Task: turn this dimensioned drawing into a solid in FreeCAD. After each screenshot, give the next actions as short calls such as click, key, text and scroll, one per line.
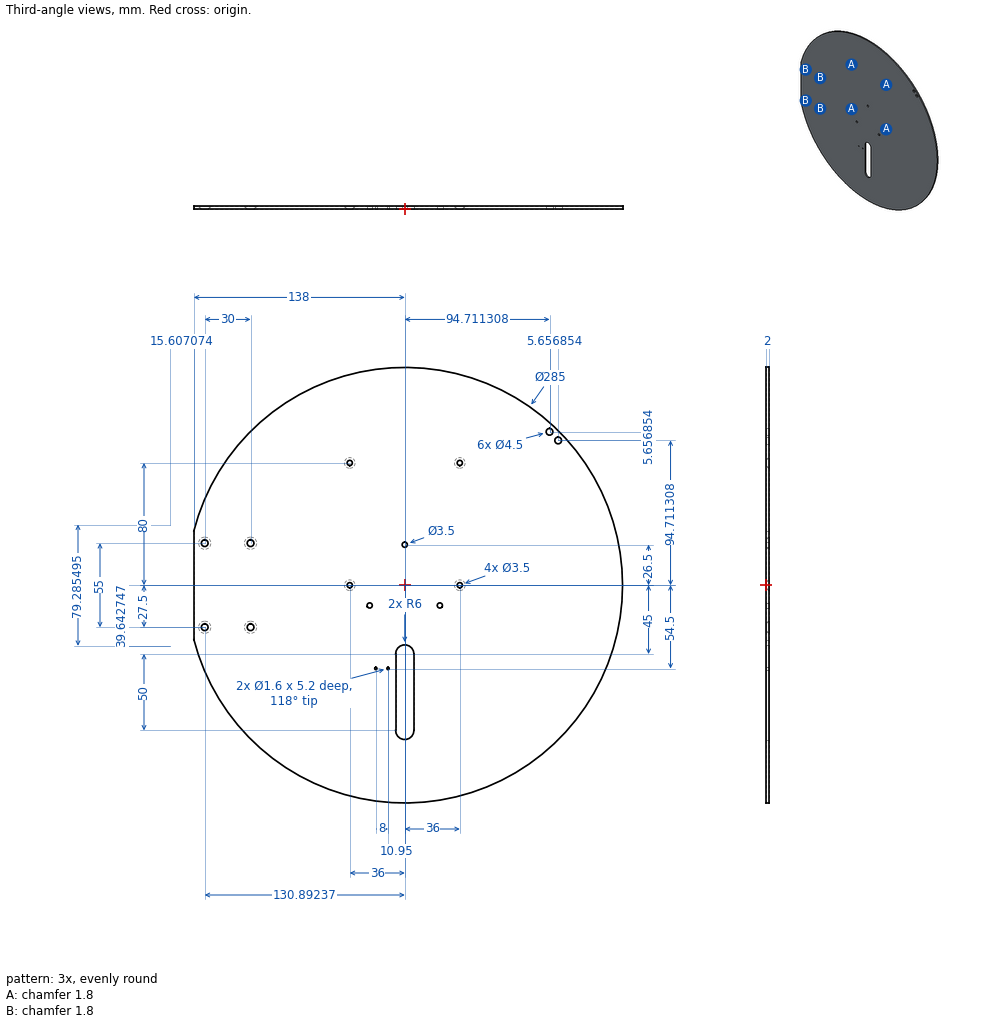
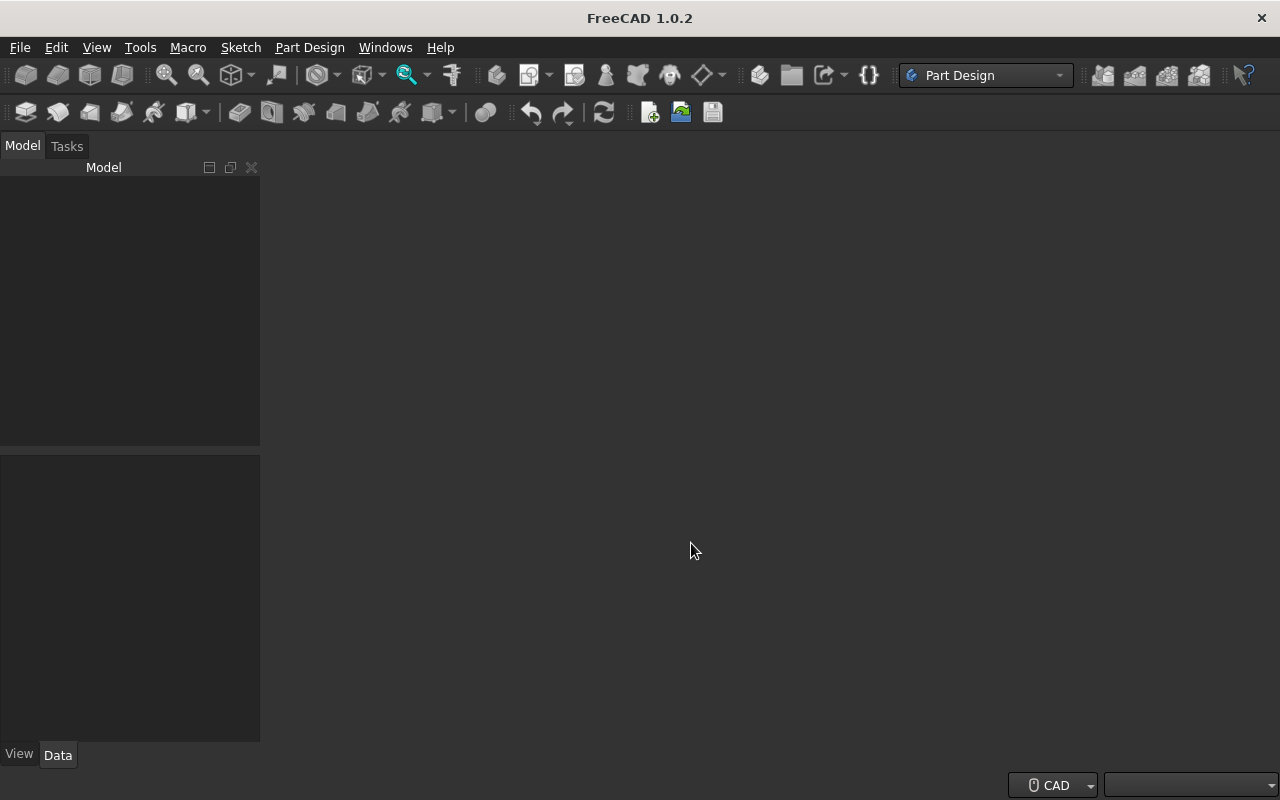
click(650, 112)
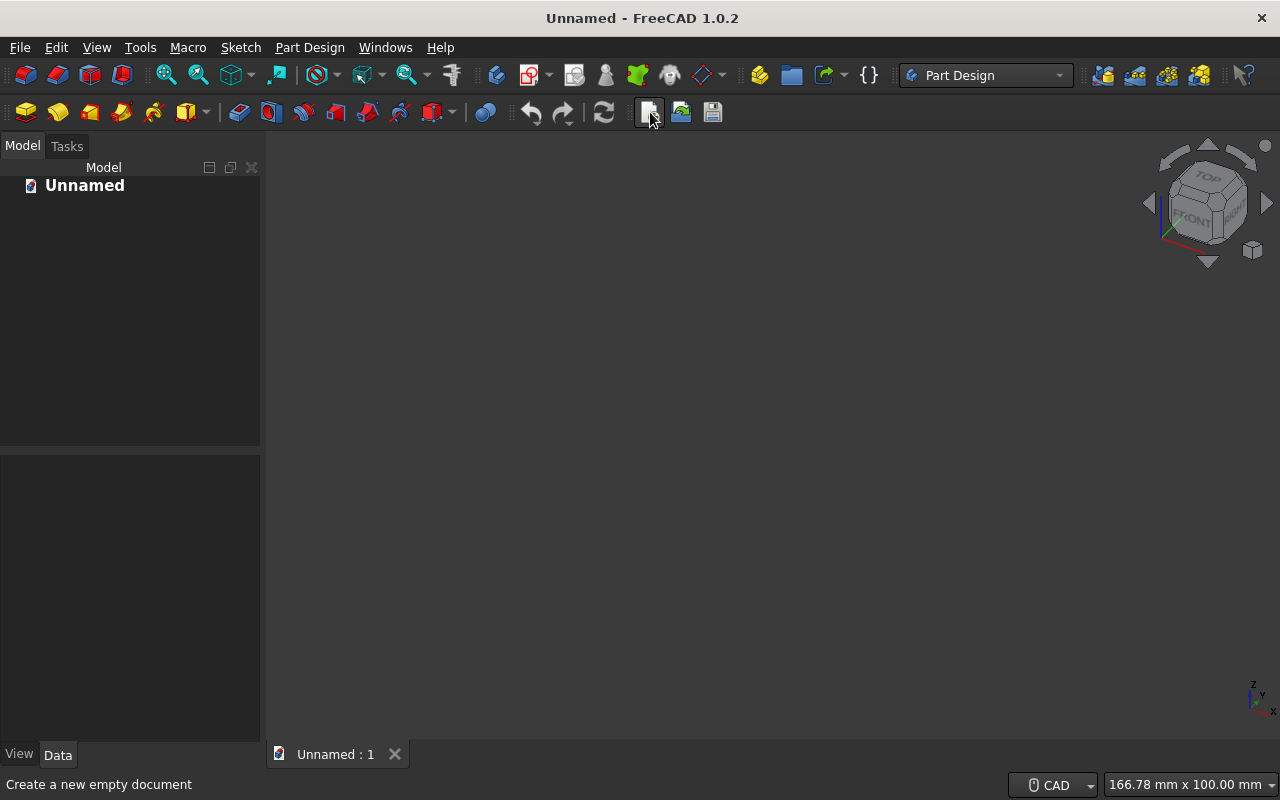
click(530, 76)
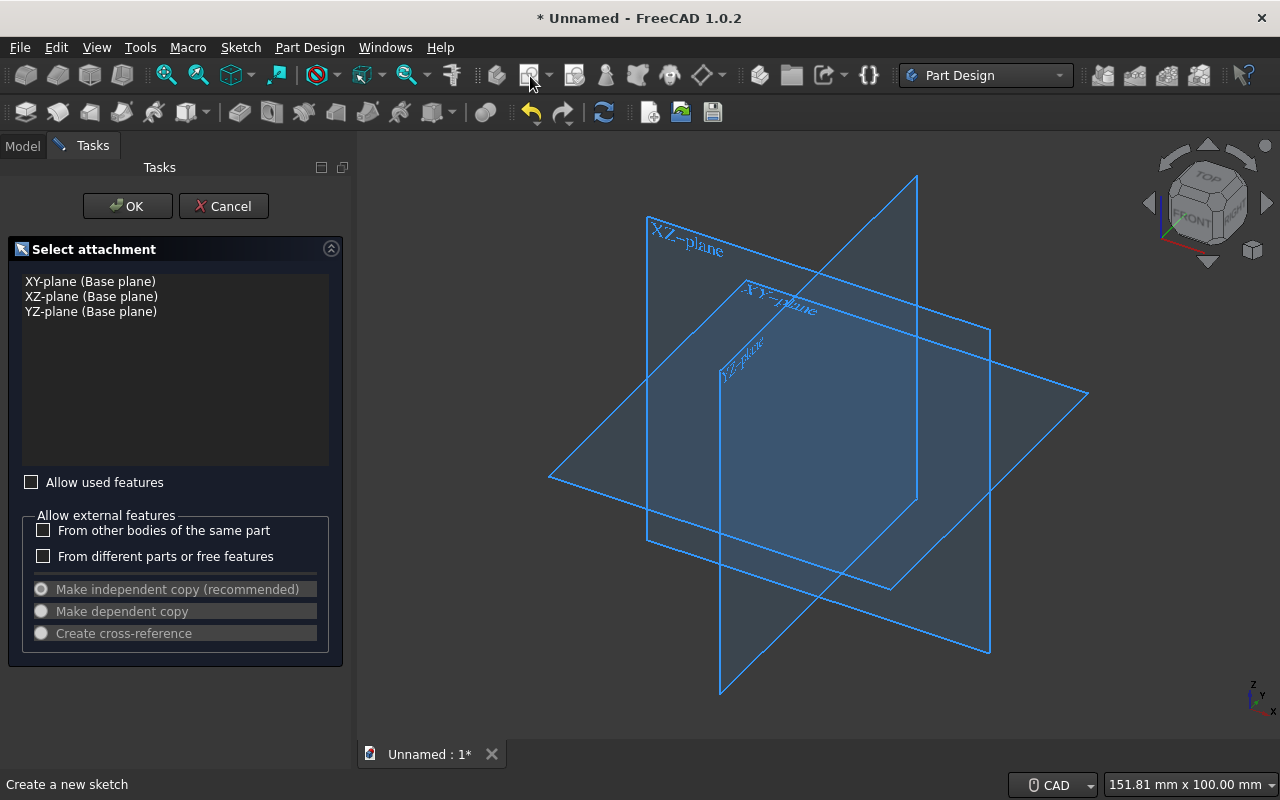
click(82, 296)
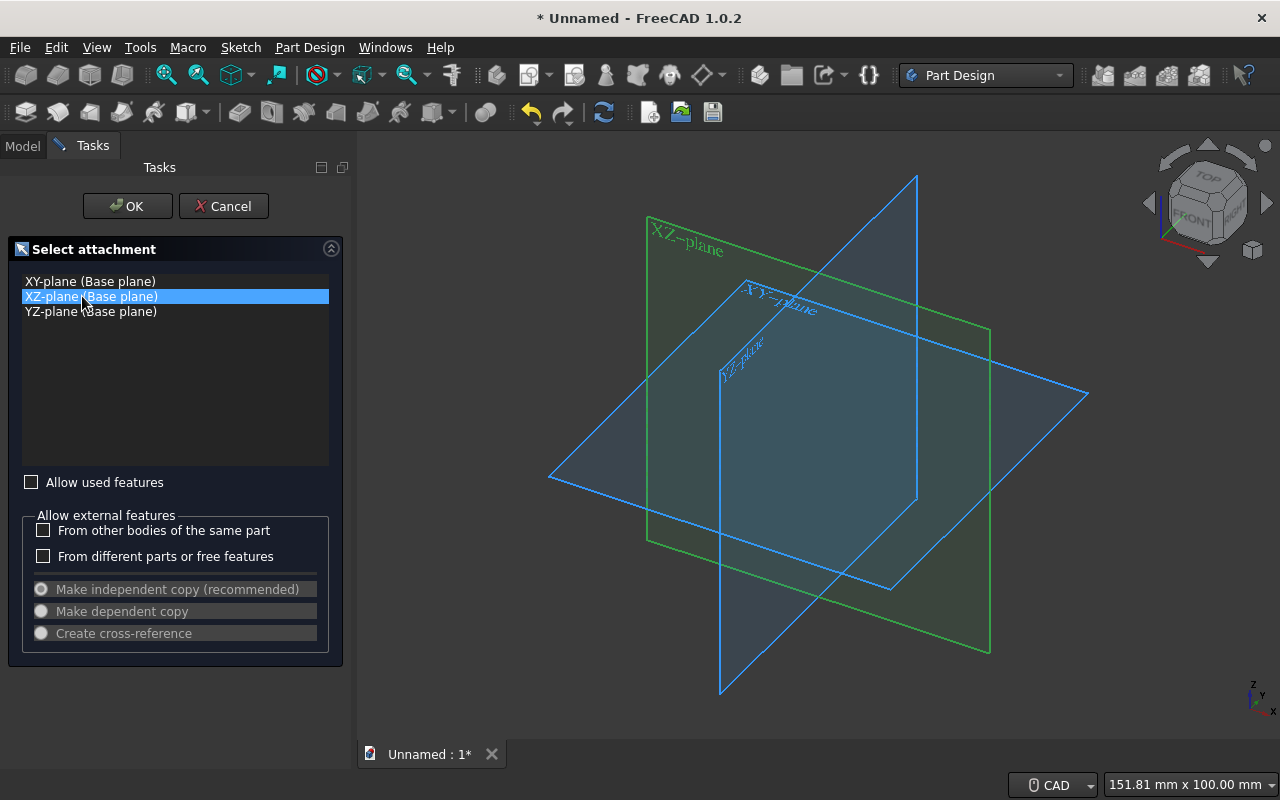
click(128, 206)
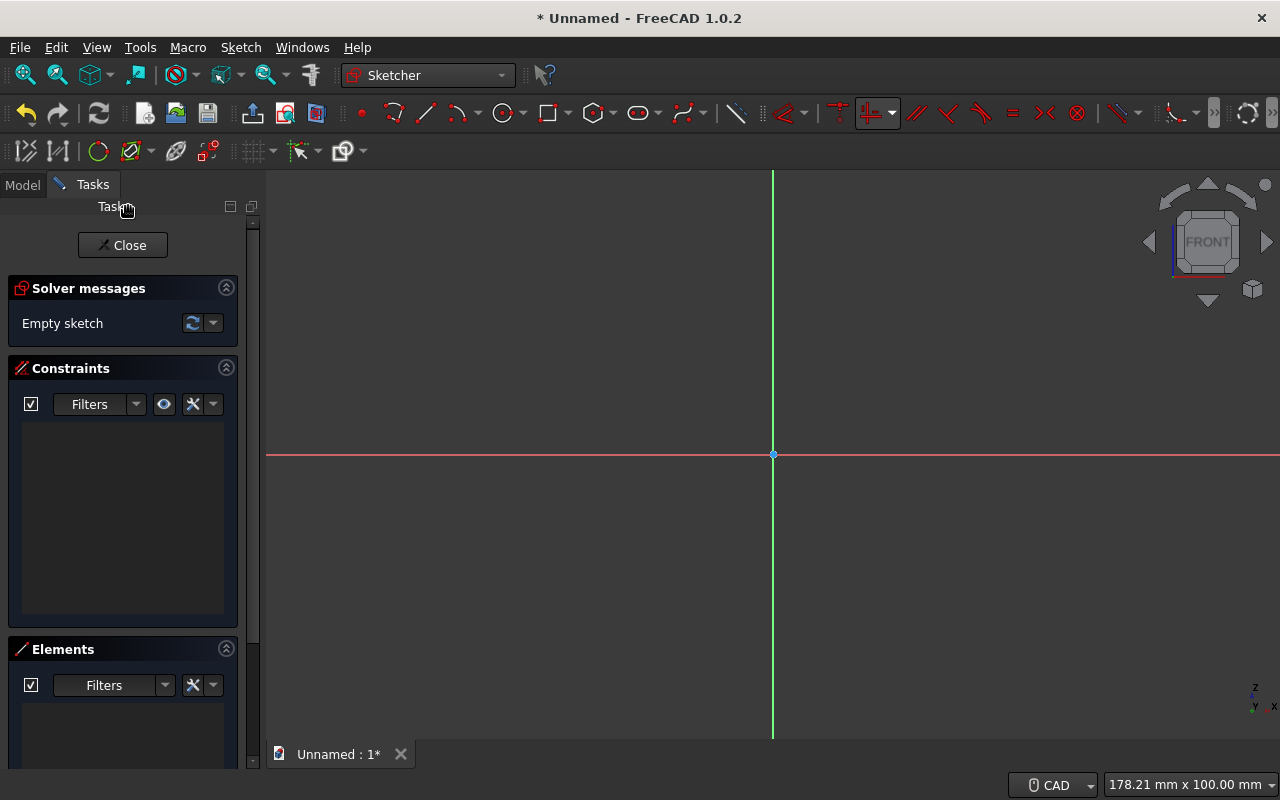
scroll(682, 454, down, 7)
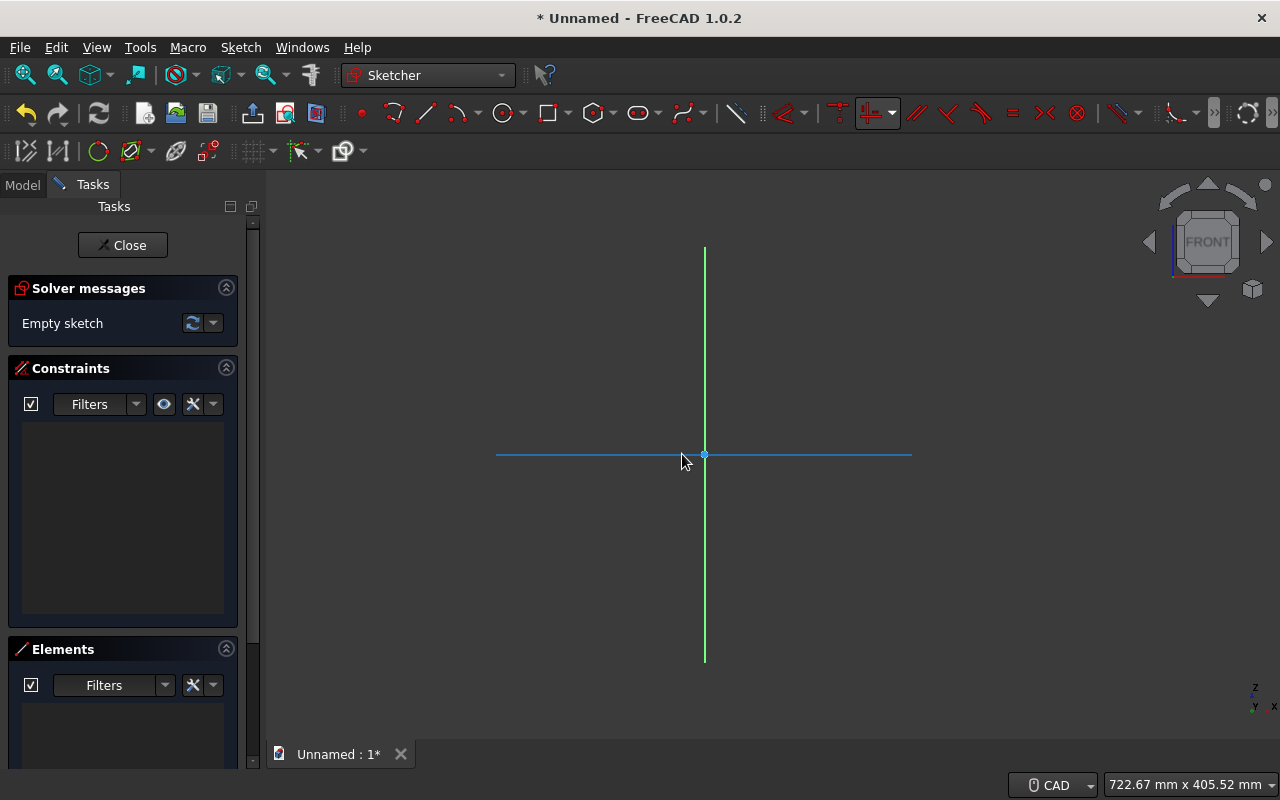
click(504, 114)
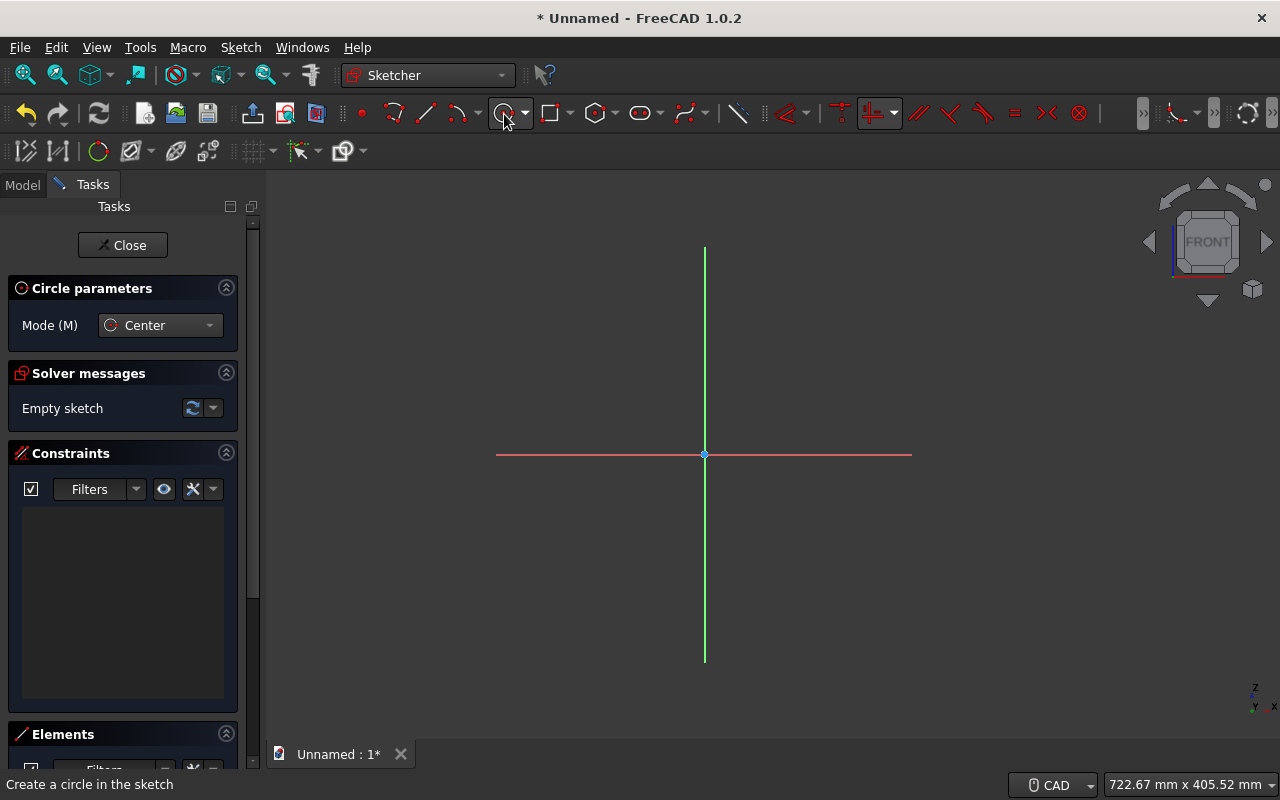
click(705, 454)
click(846, 313)
key(Escape)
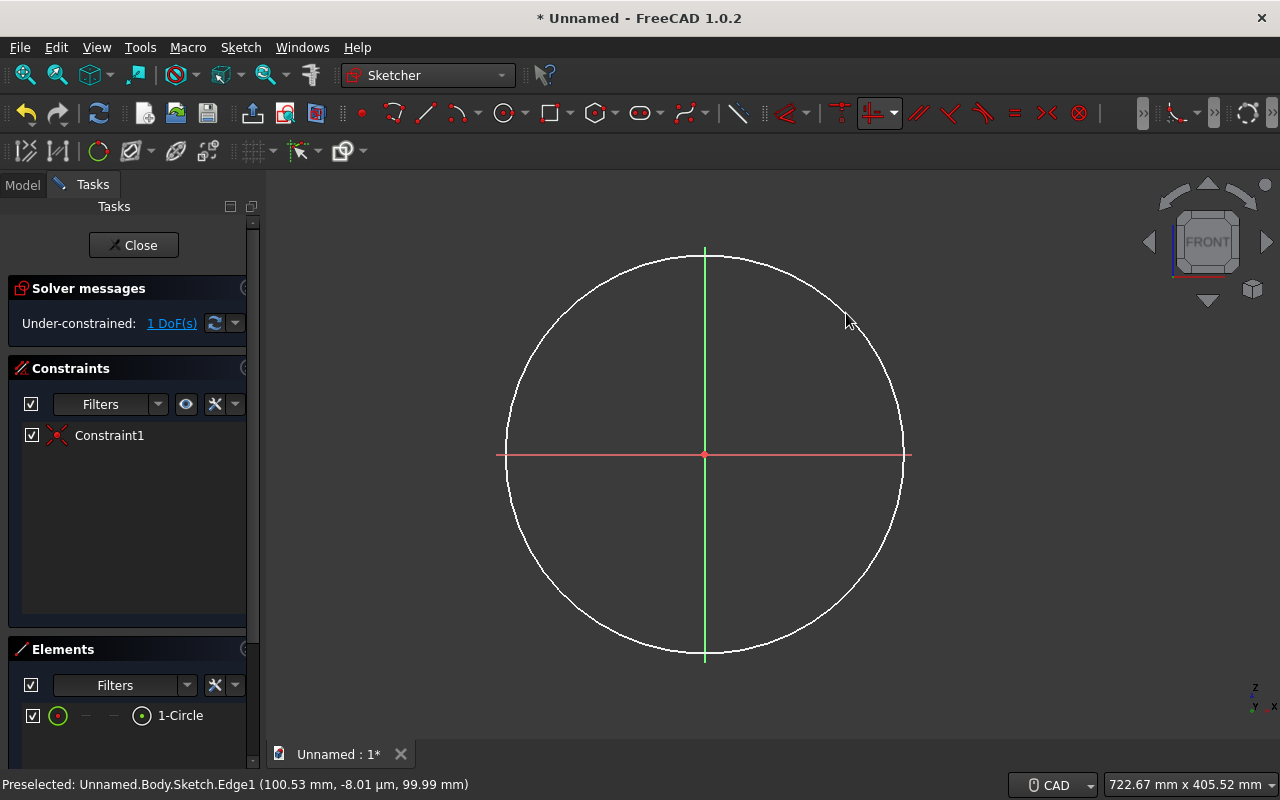
click(786, 114)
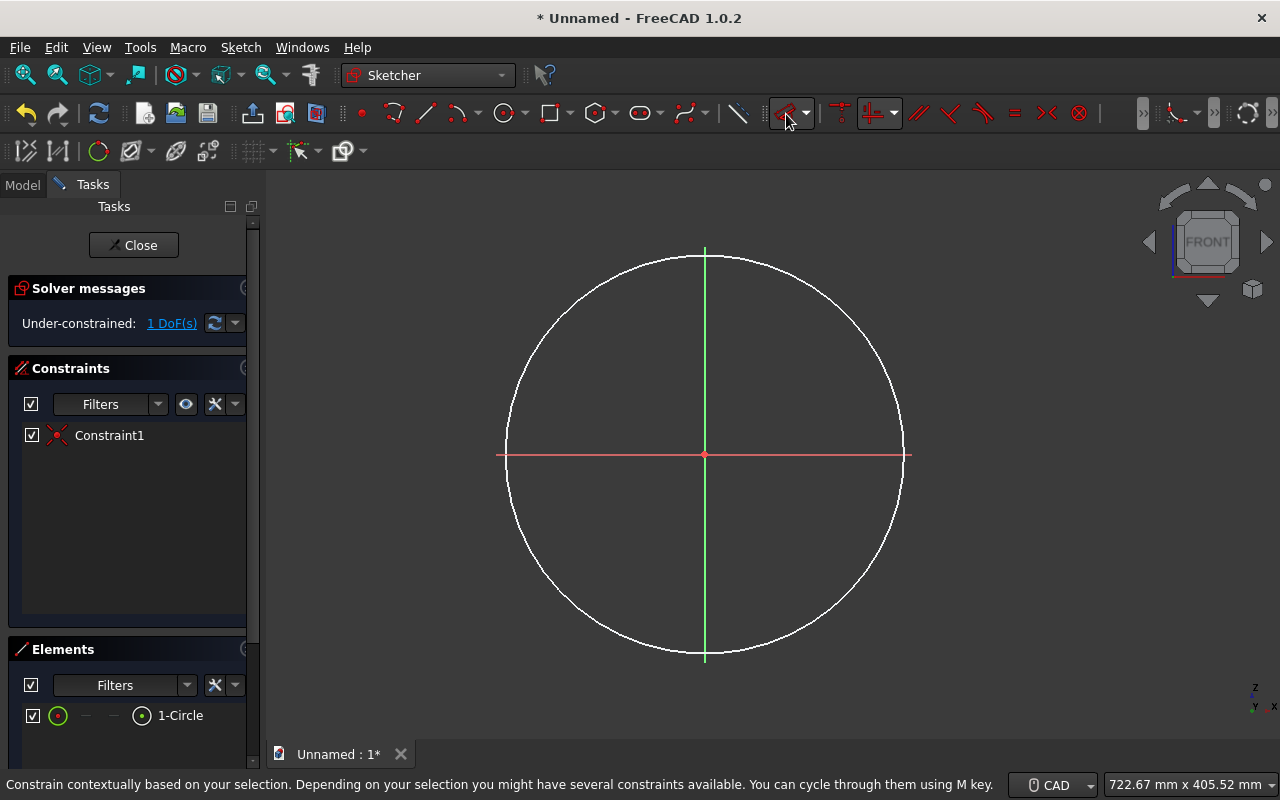
click(845, 313)
click(868, 290)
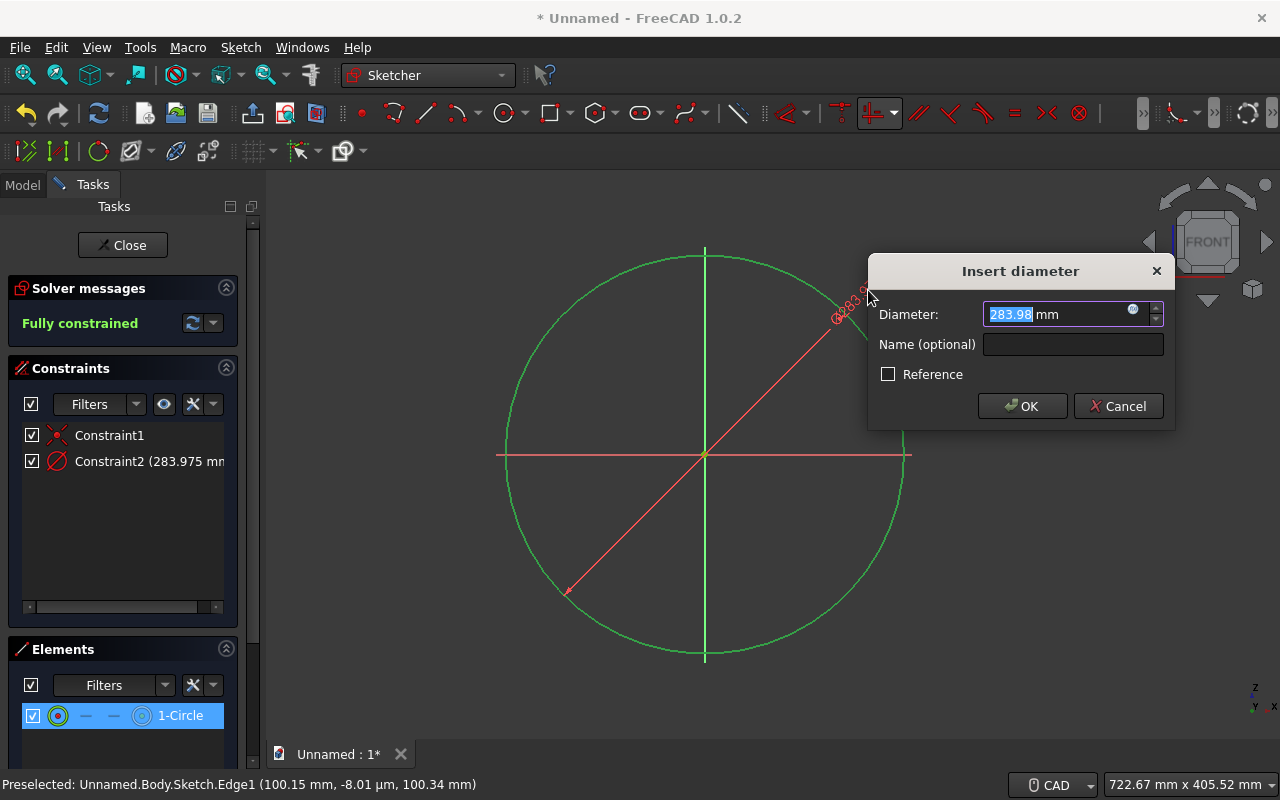
text(285)
key(Return)
key(Escape)